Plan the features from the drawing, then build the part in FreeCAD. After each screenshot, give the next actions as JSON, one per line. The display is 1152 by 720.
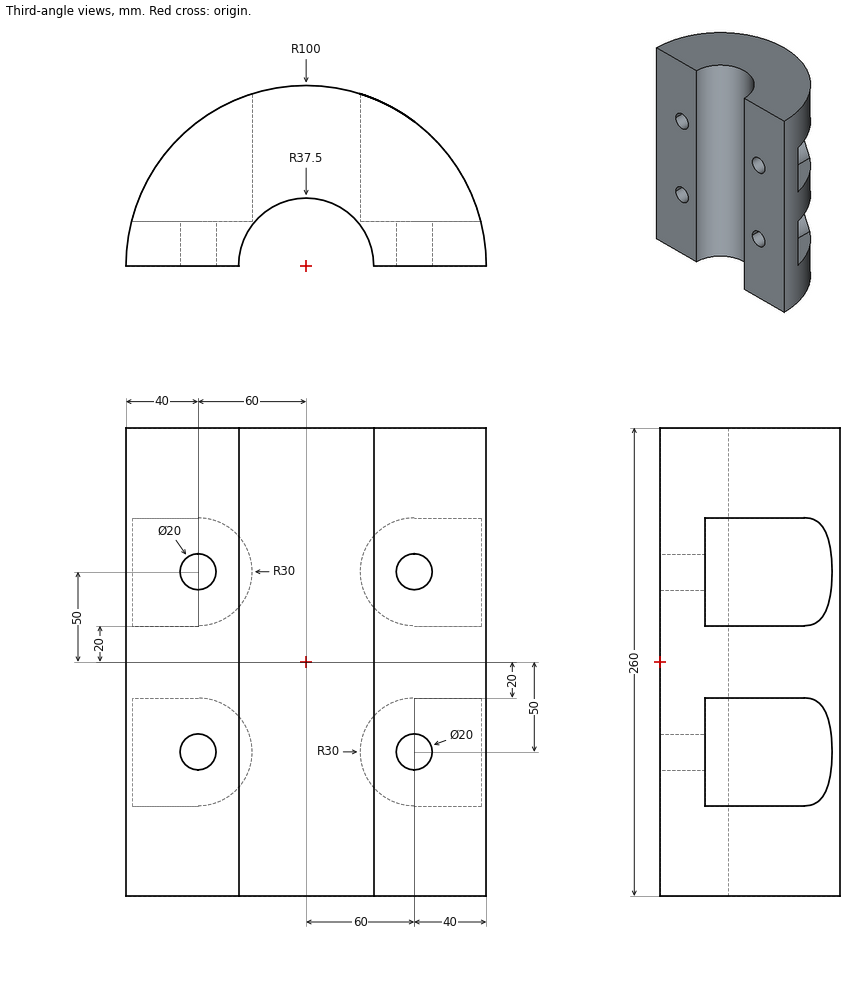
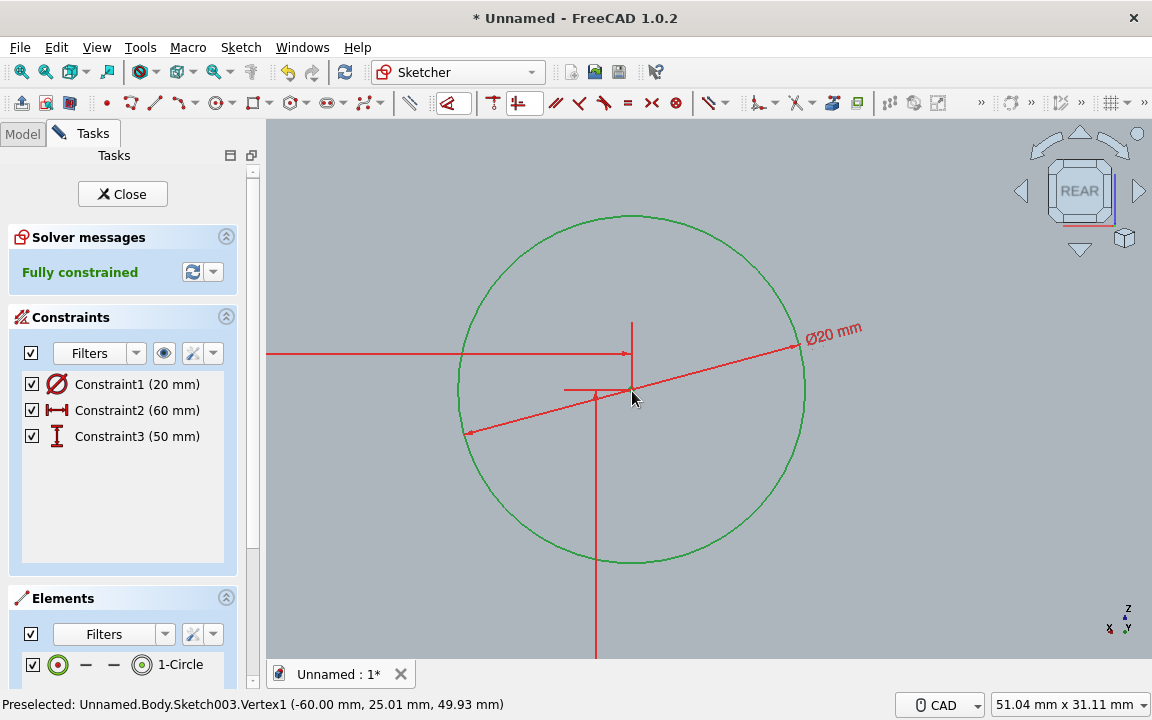
{"action": "left_click", "coordinate": [123, 194]}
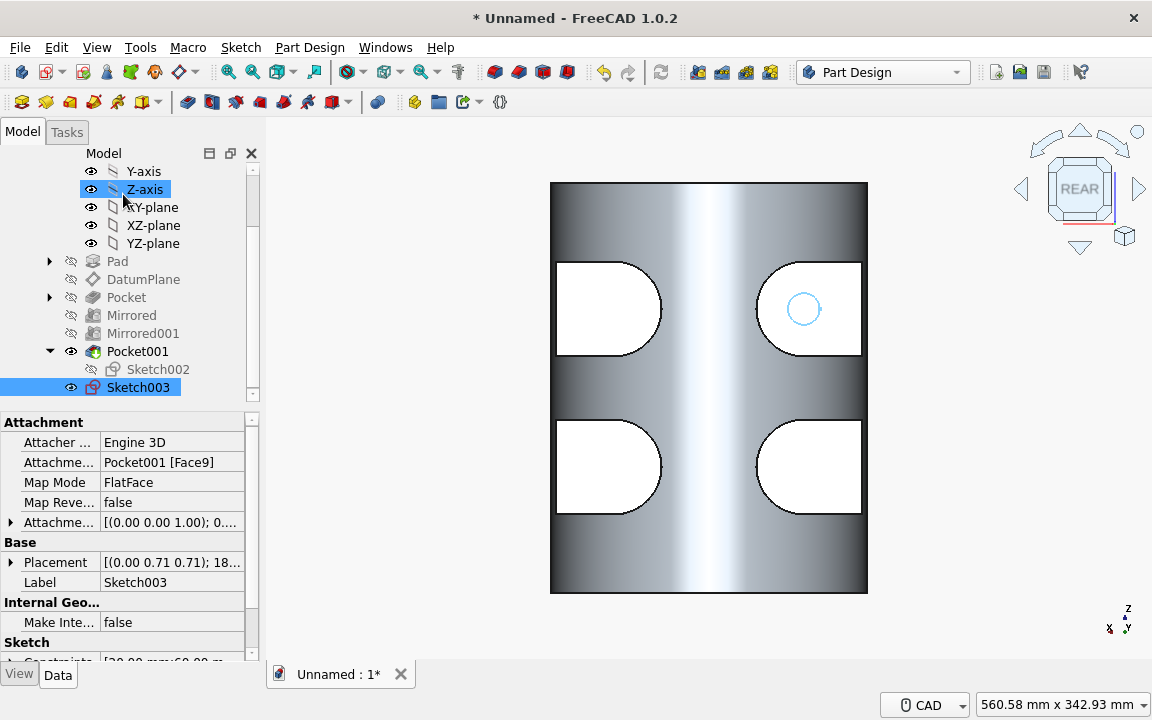
{"action": "left_click", "coordinate": [188, 102]}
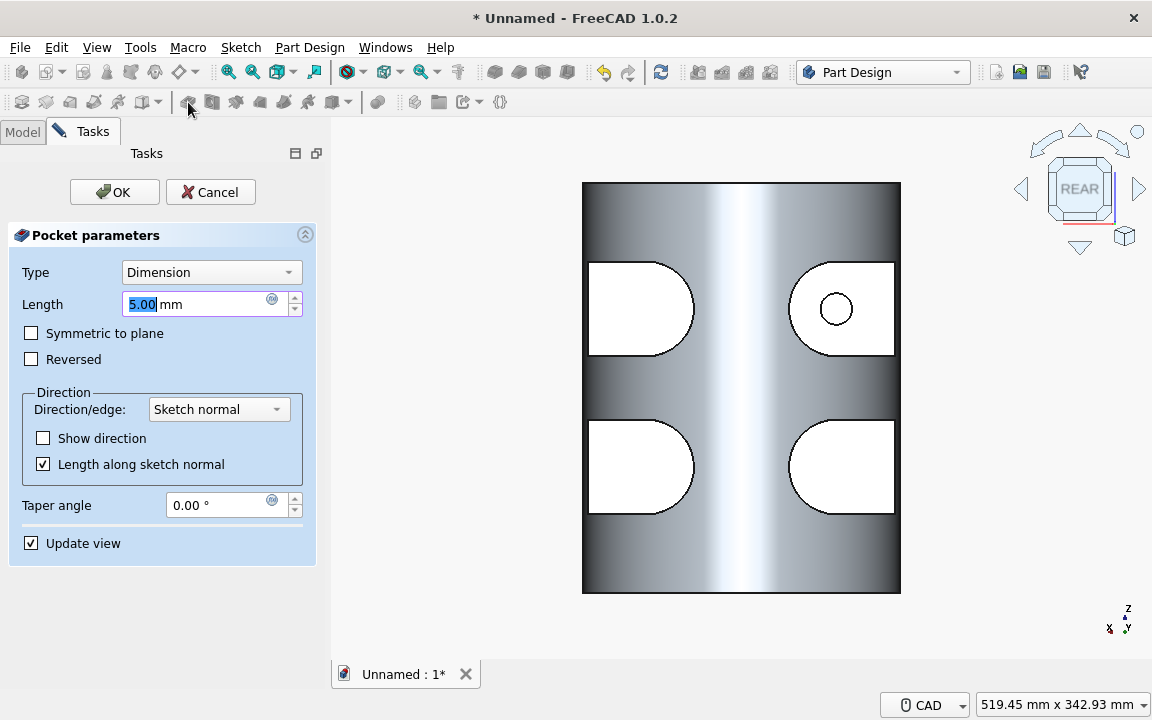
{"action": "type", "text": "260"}
{"action": "key", "text": "Tab"}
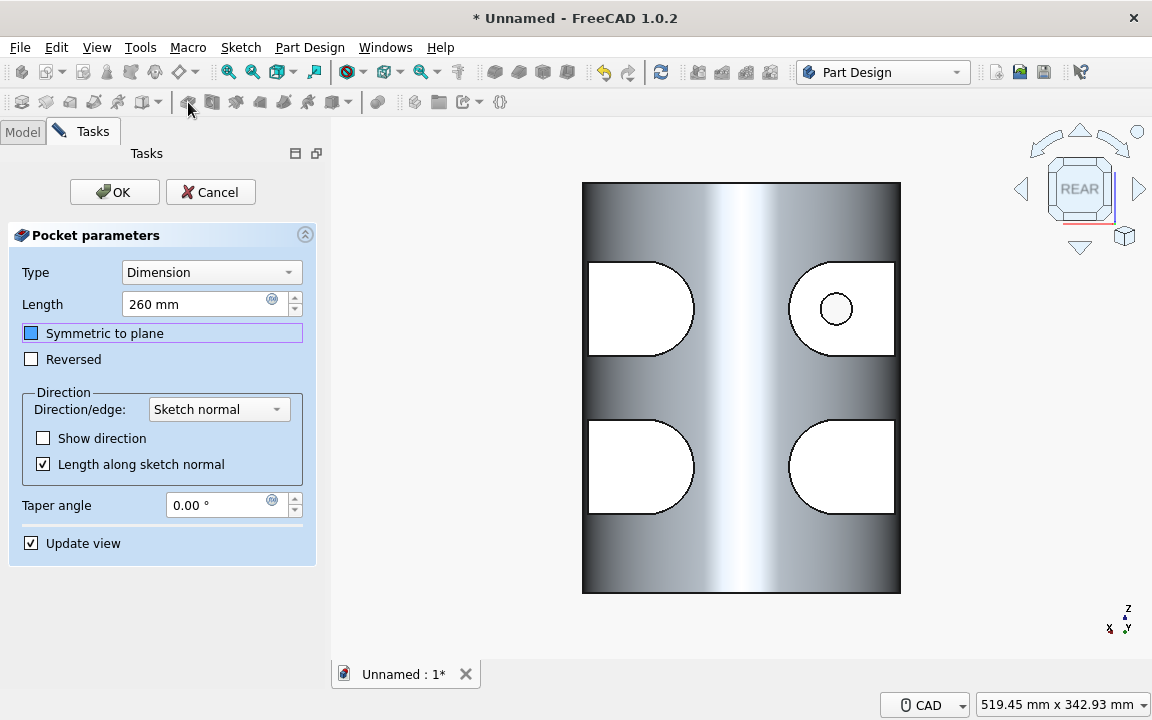
{"action": "left_click", "coordinate": [115, 192]}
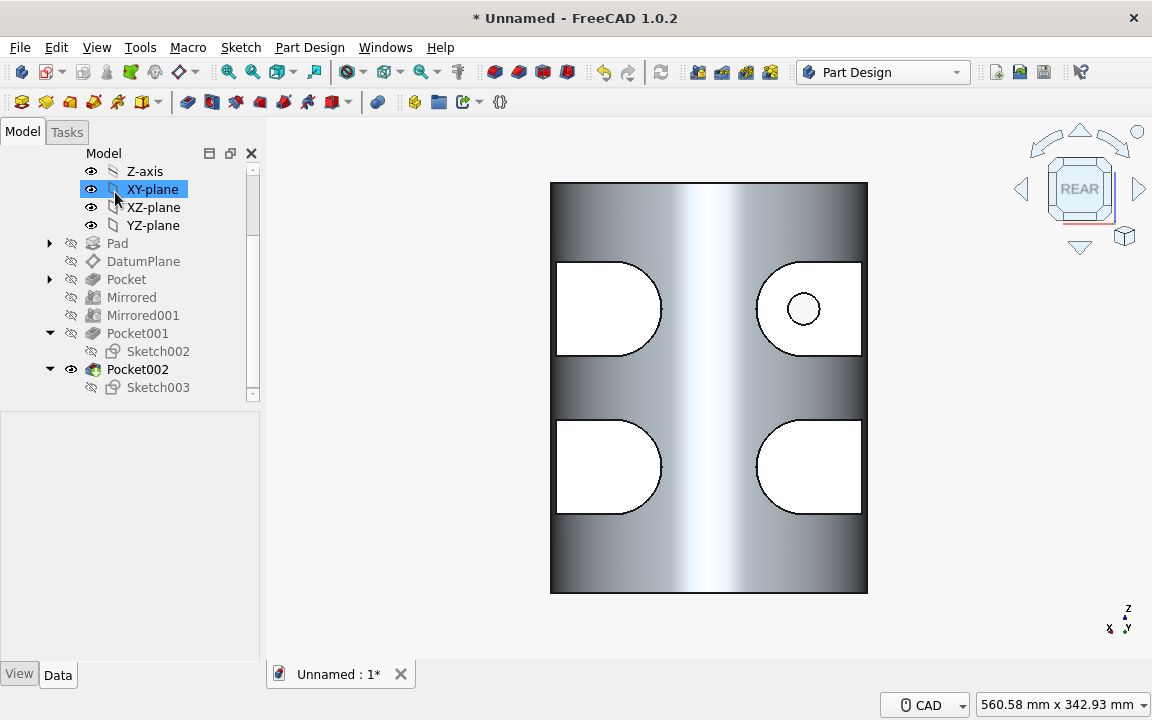
{"action": "left_click", "coordinate": [116, 369]}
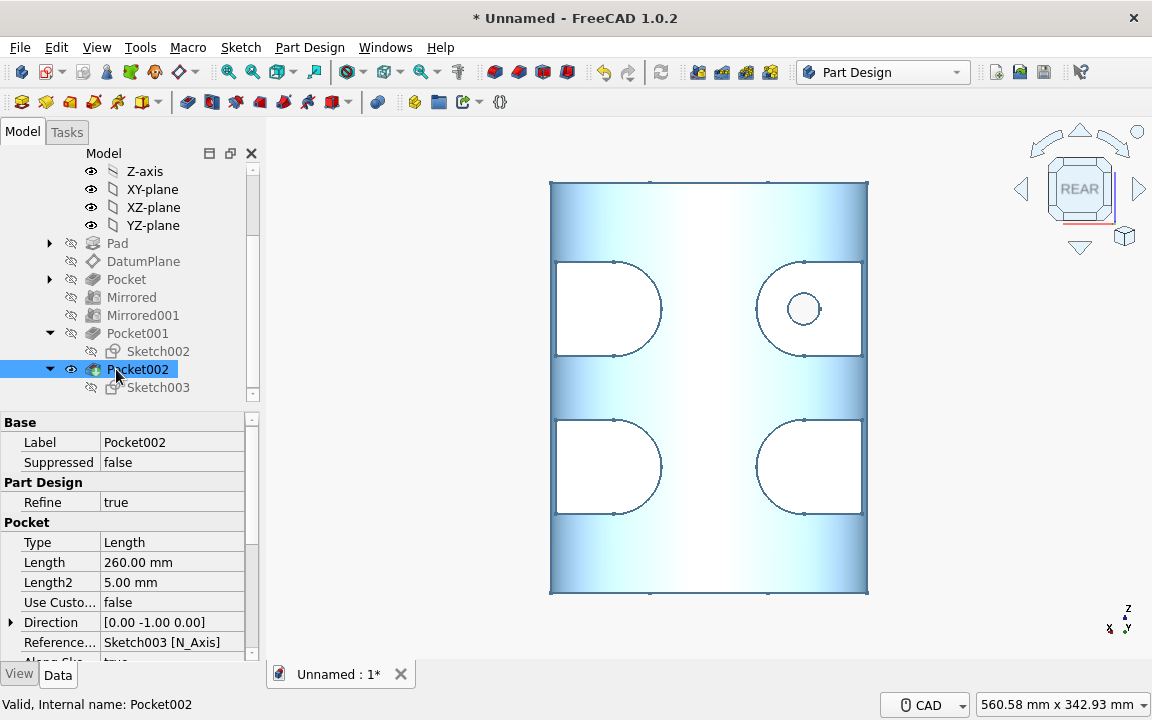
{"action": "left_click", "coordinate": [698, 72]}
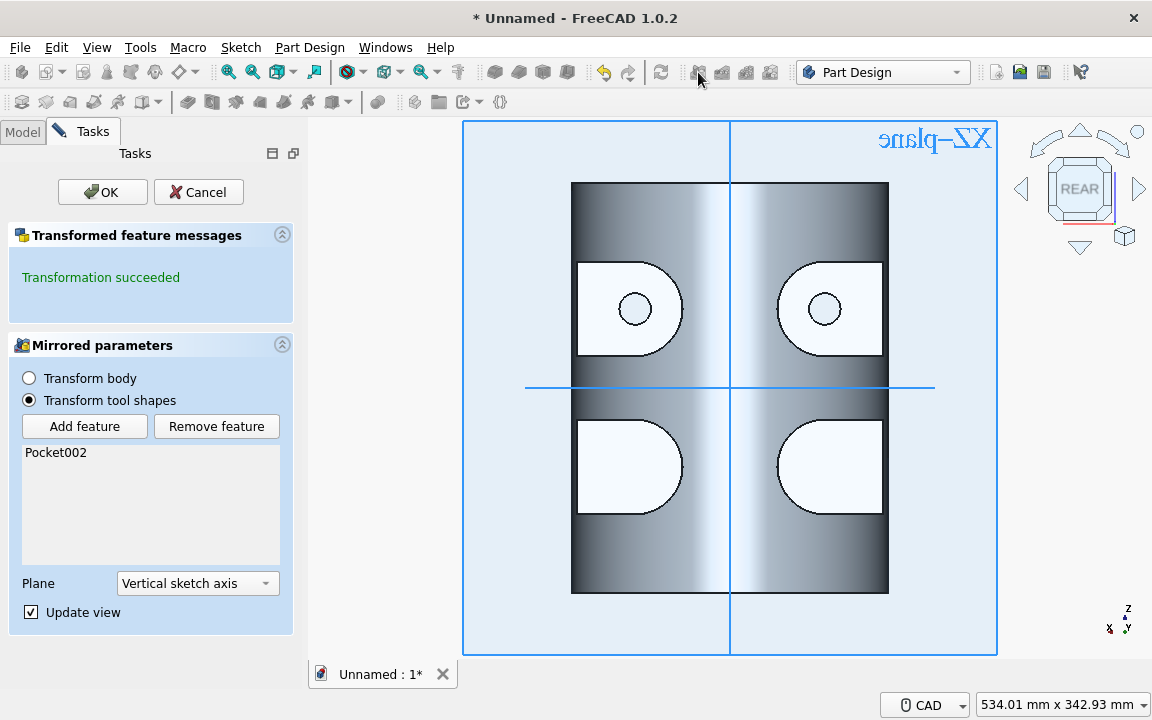
{"action": "left_click", "coordinate": [198, 584]}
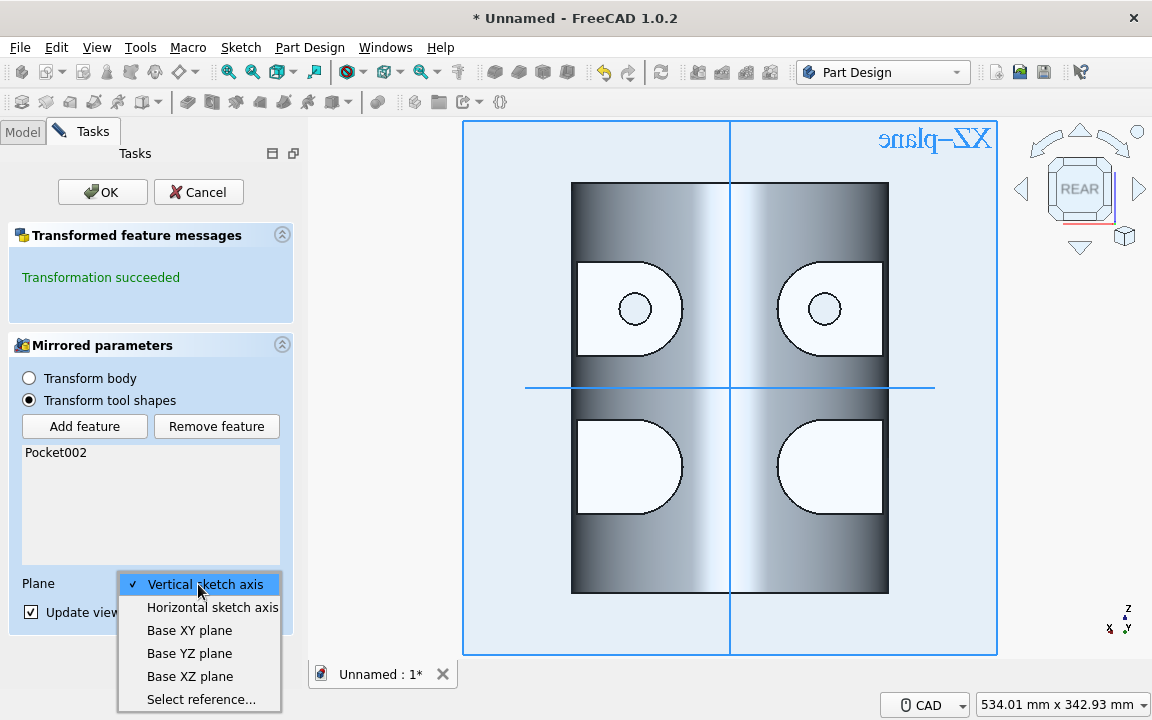
{"action": "left_click", "coordinate": [198, 630]}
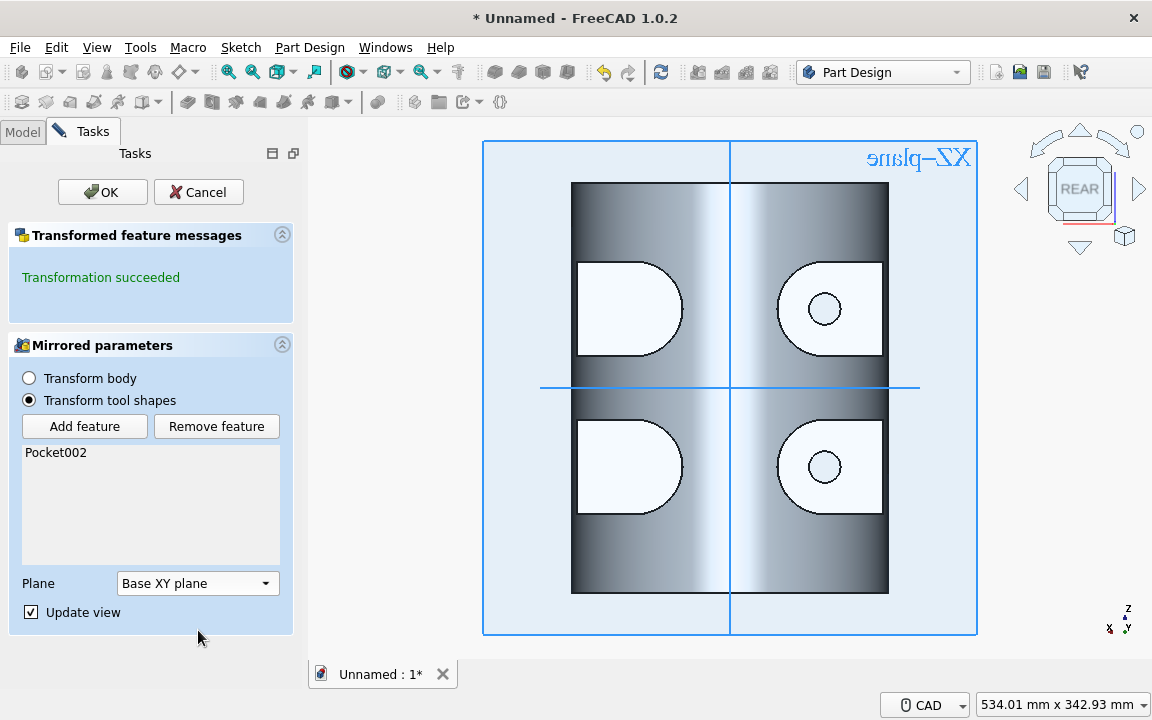
{"action": "left_click", "coordinate": [103, 192]}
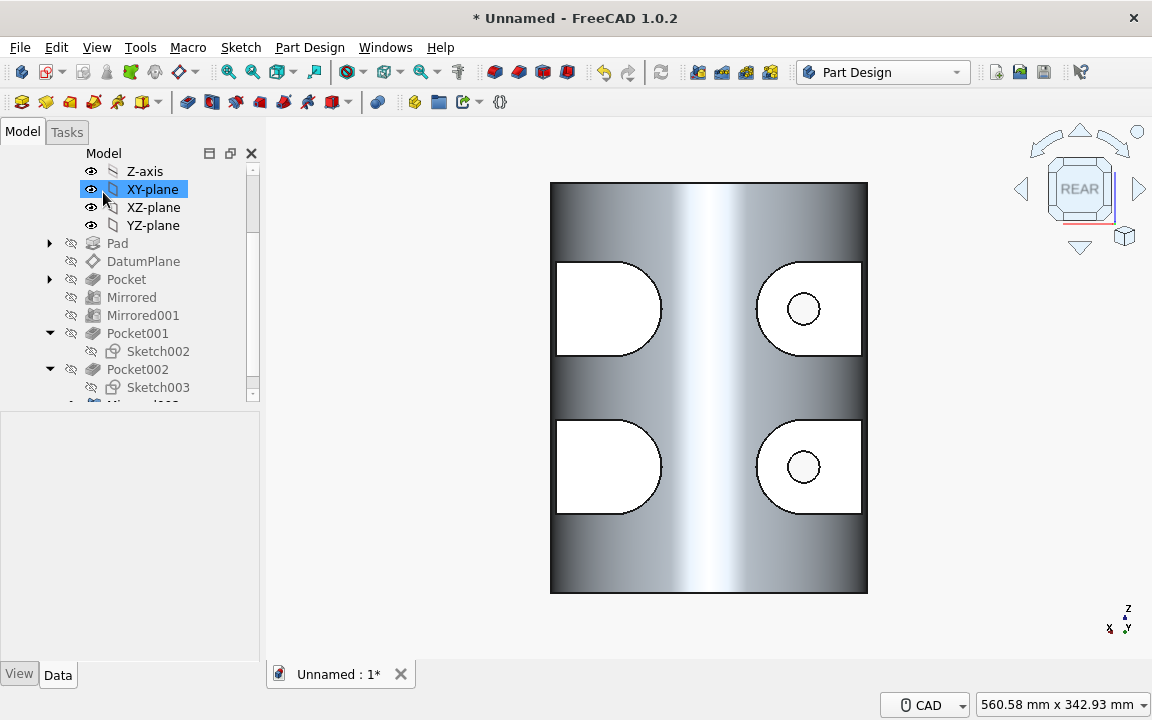
{"action": "left_click", "coordinate": [116, 369]}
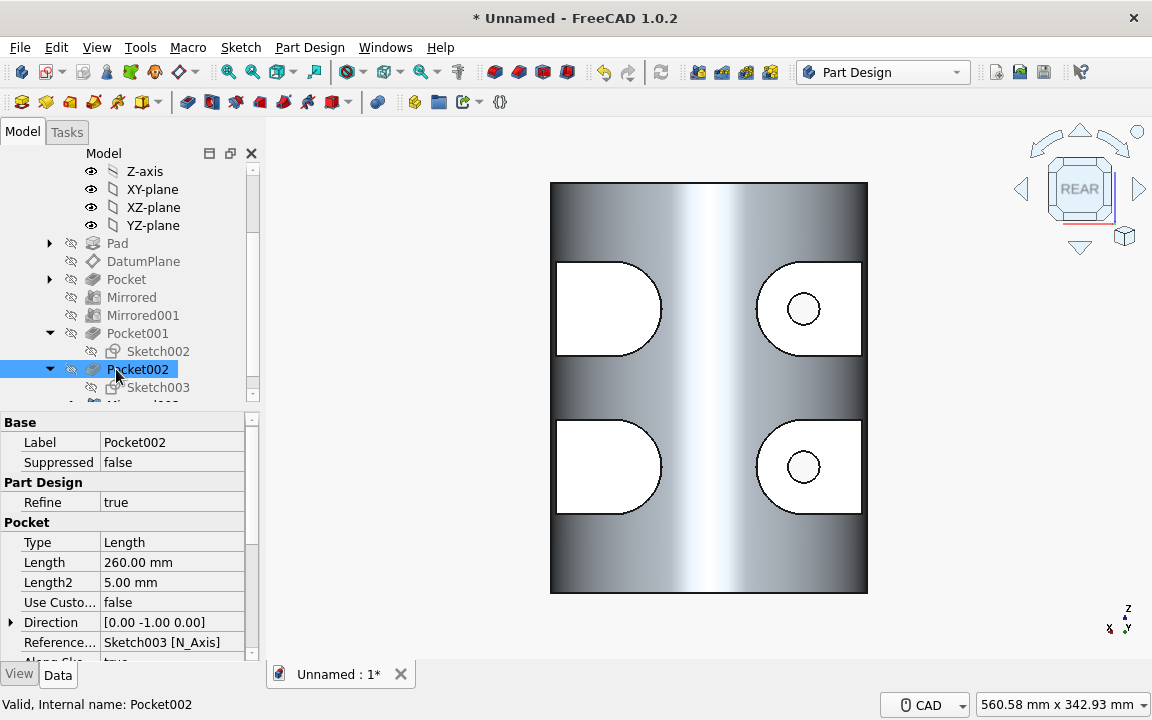
{"action": "left_click", "coordinate": [698, 72]}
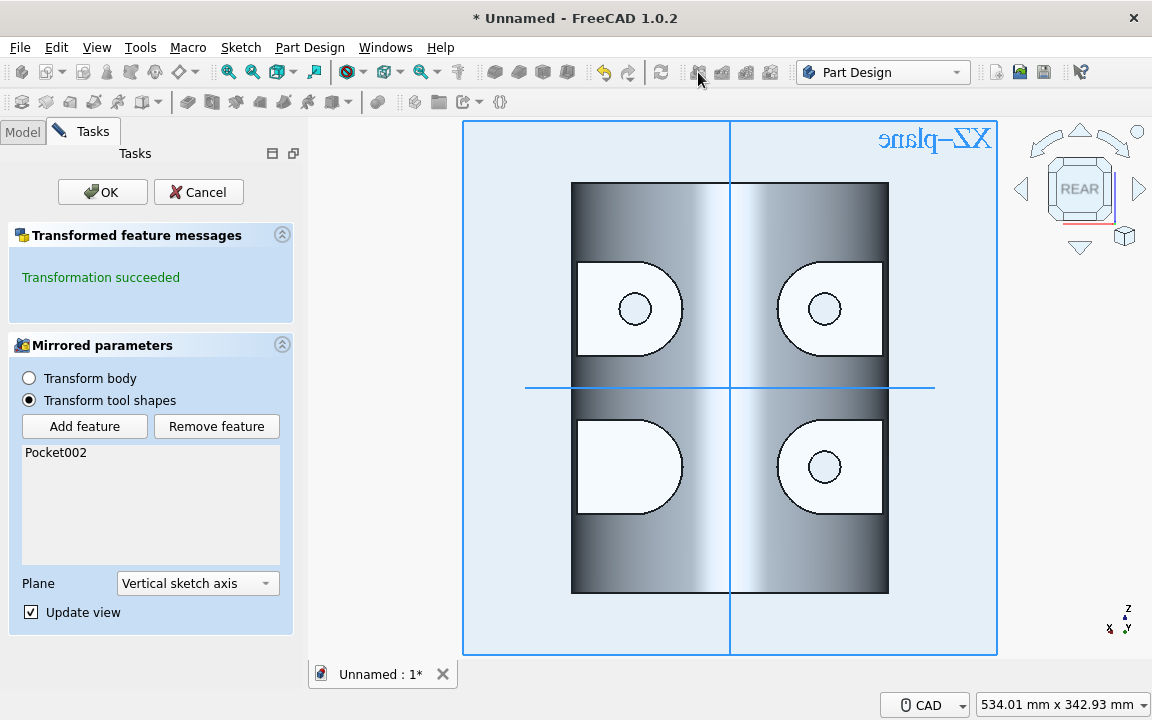
{"action": "left_click", "coordinate": [198, 584]}